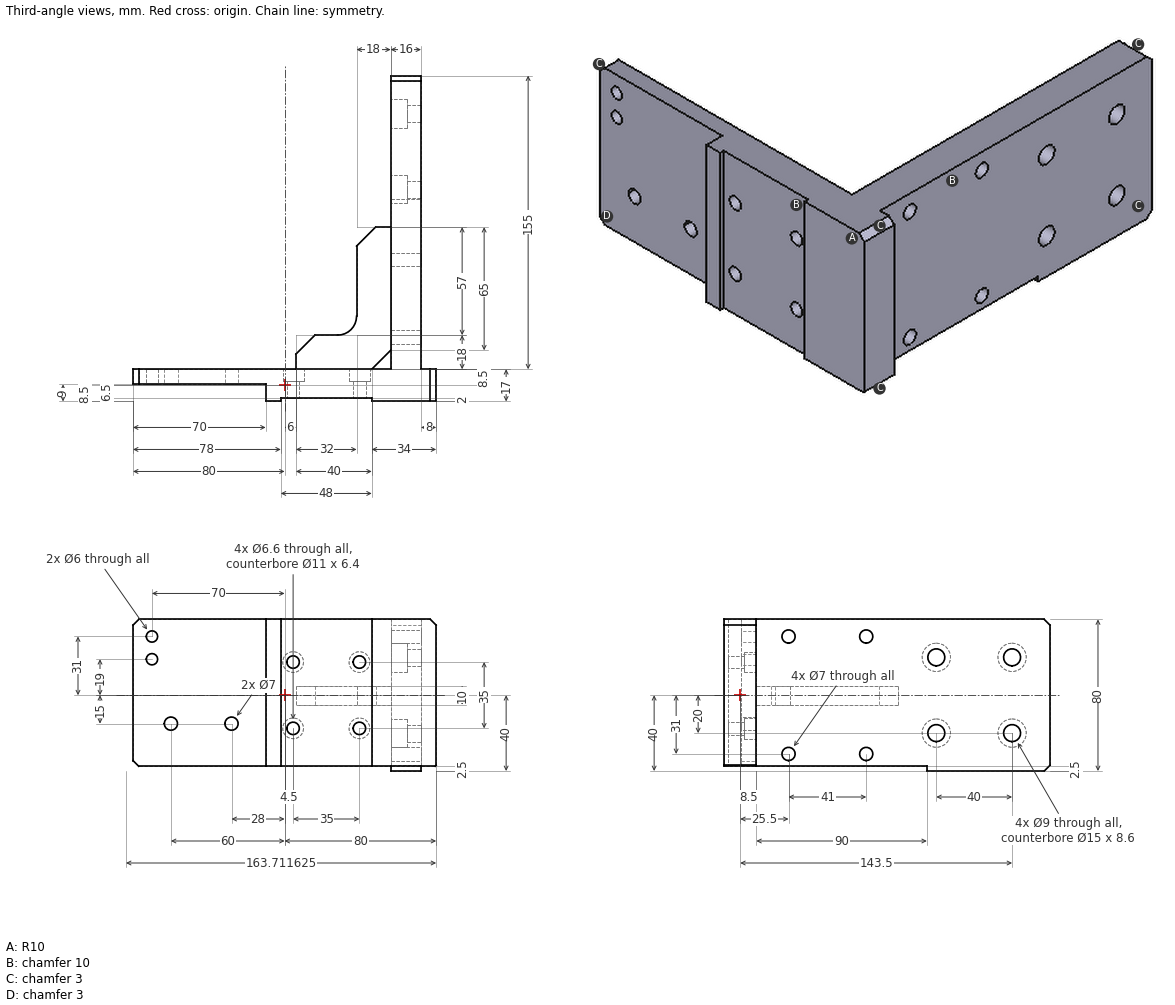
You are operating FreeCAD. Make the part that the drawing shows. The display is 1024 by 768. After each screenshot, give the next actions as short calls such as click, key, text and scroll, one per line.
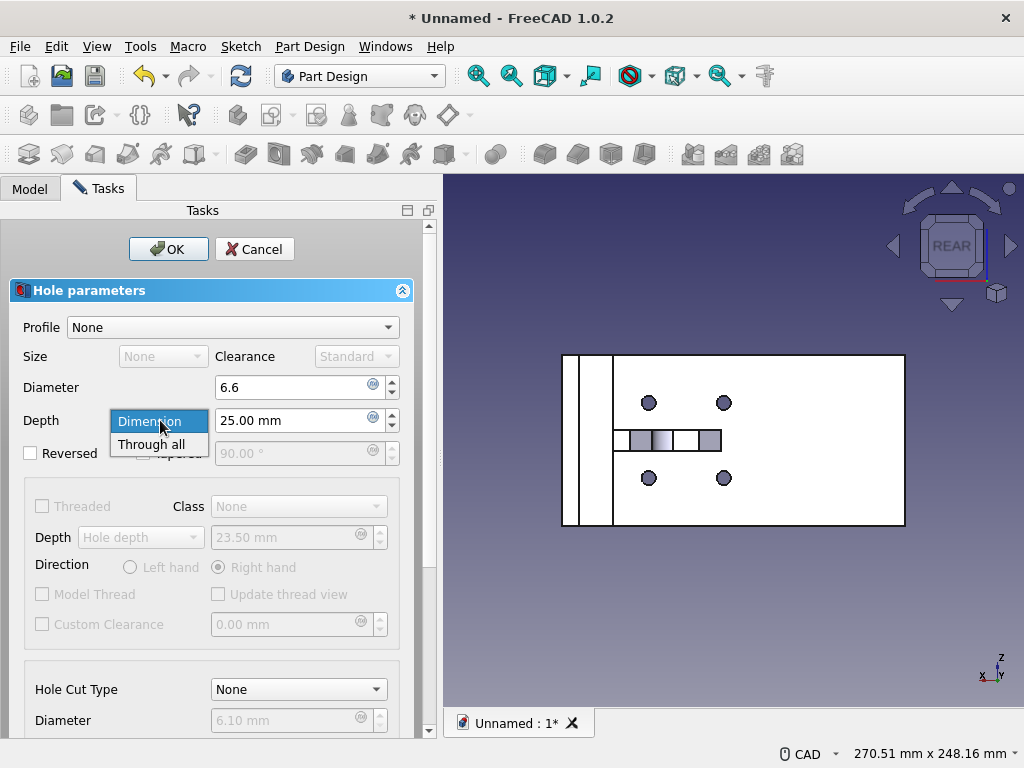
click(158, 444)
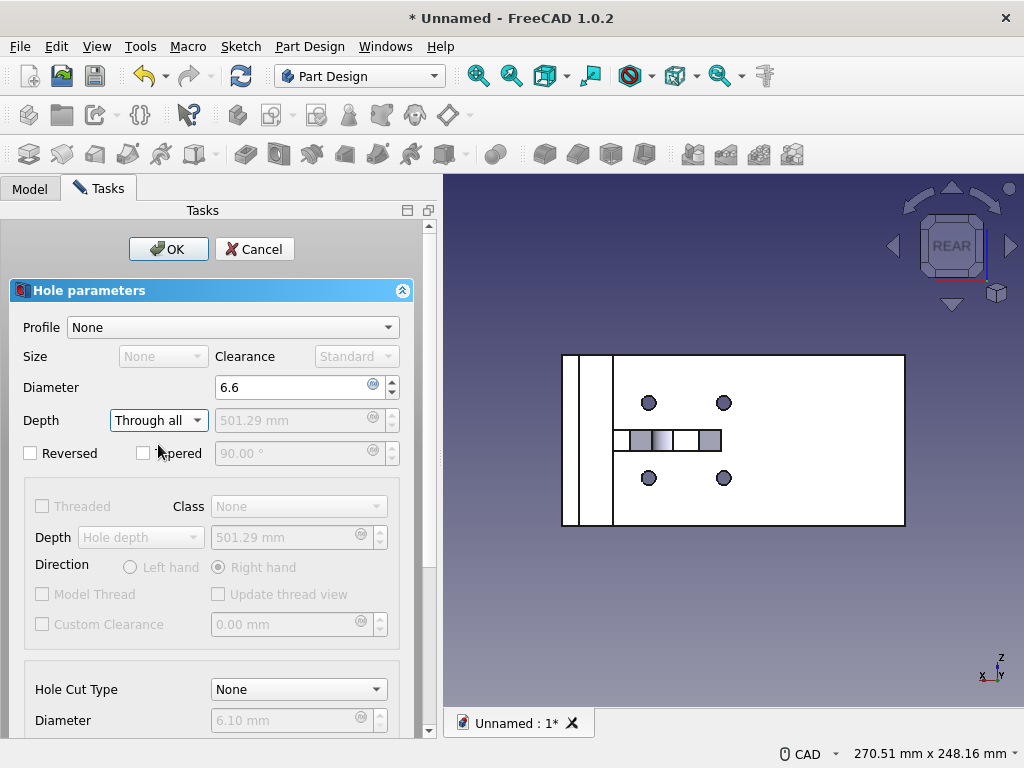
click(300, 690)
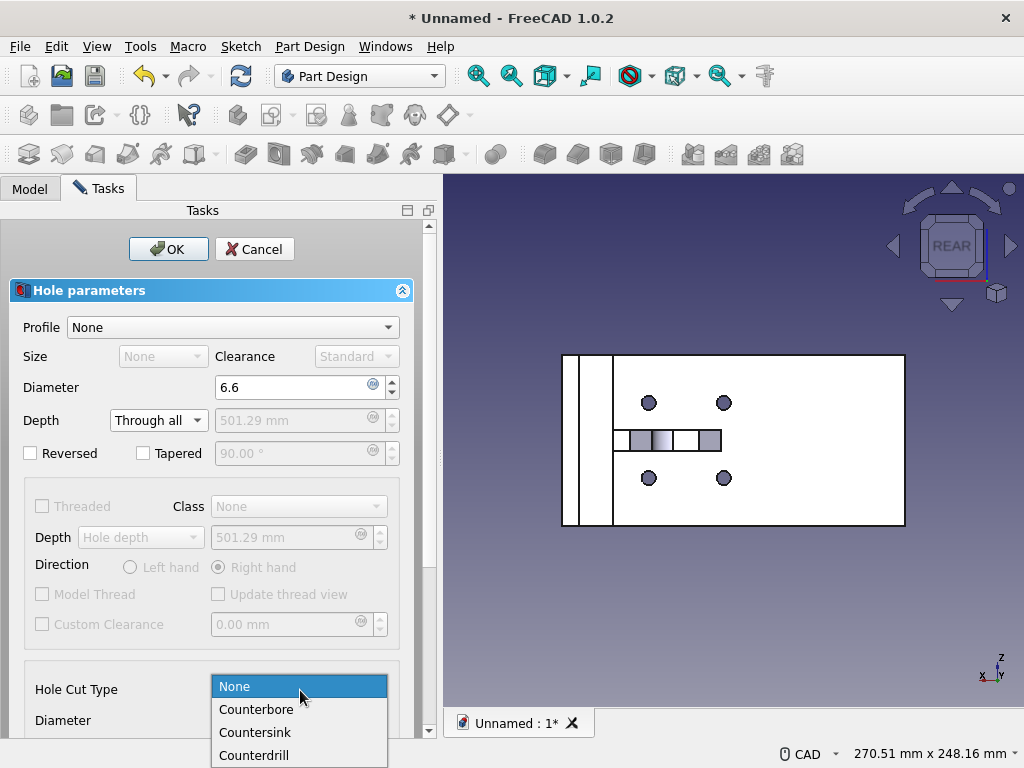
click(298, 710)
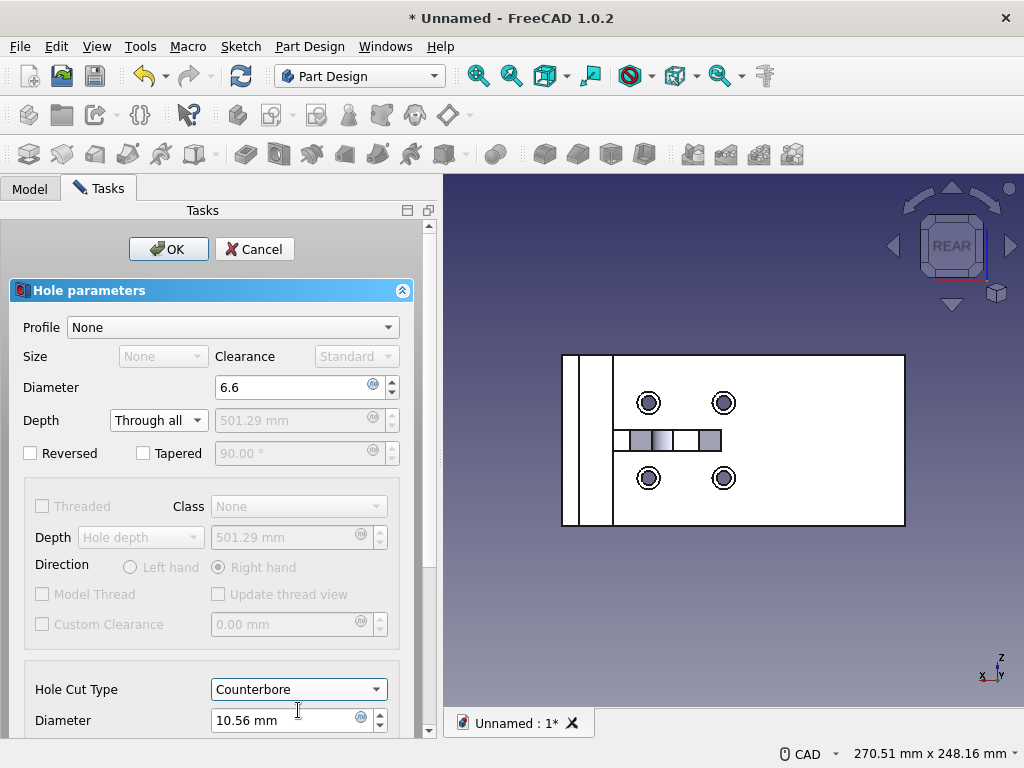
triple_click(292, 720)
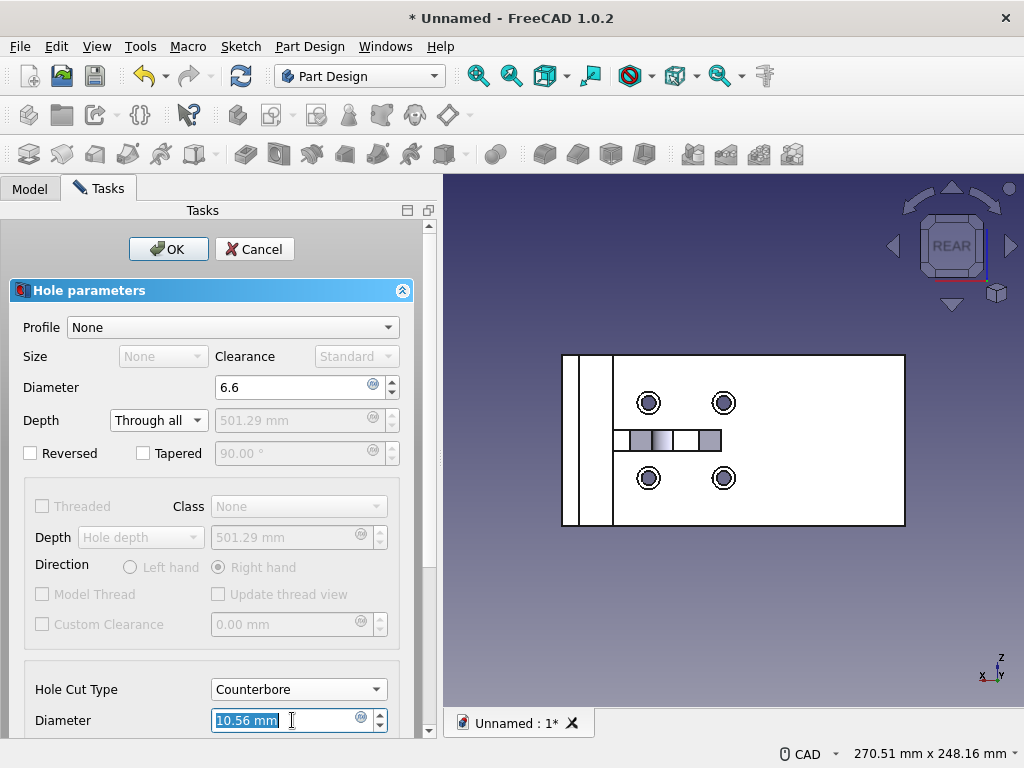
text(11)
key(Tab)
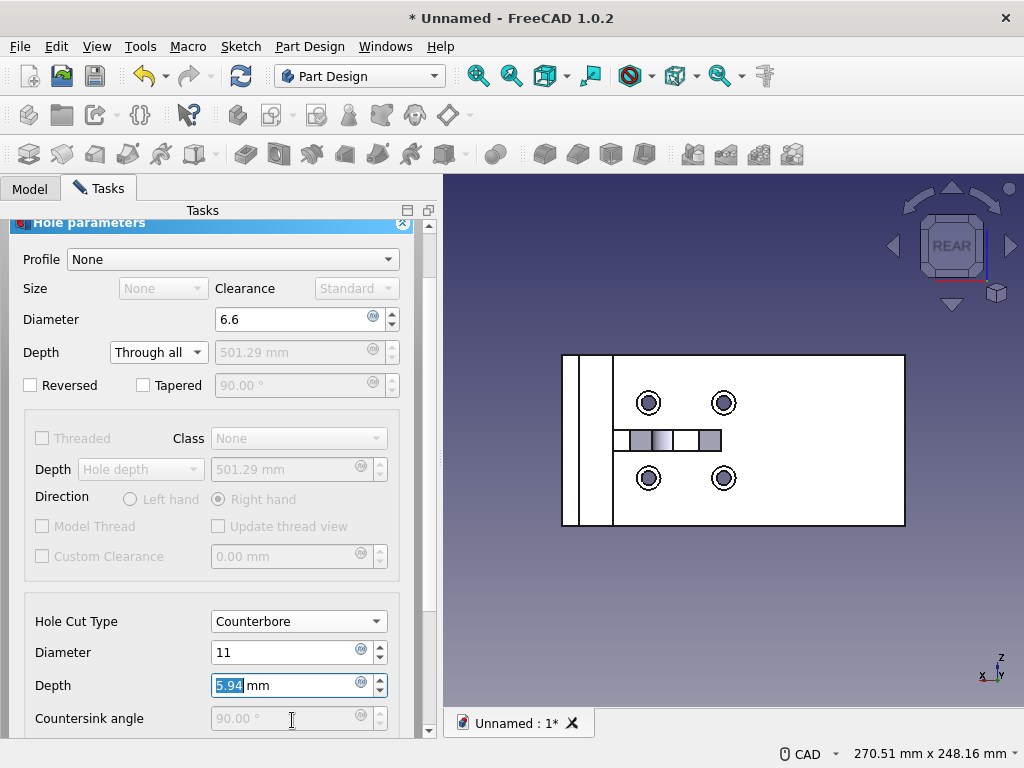
text(6.4)
key(Tab)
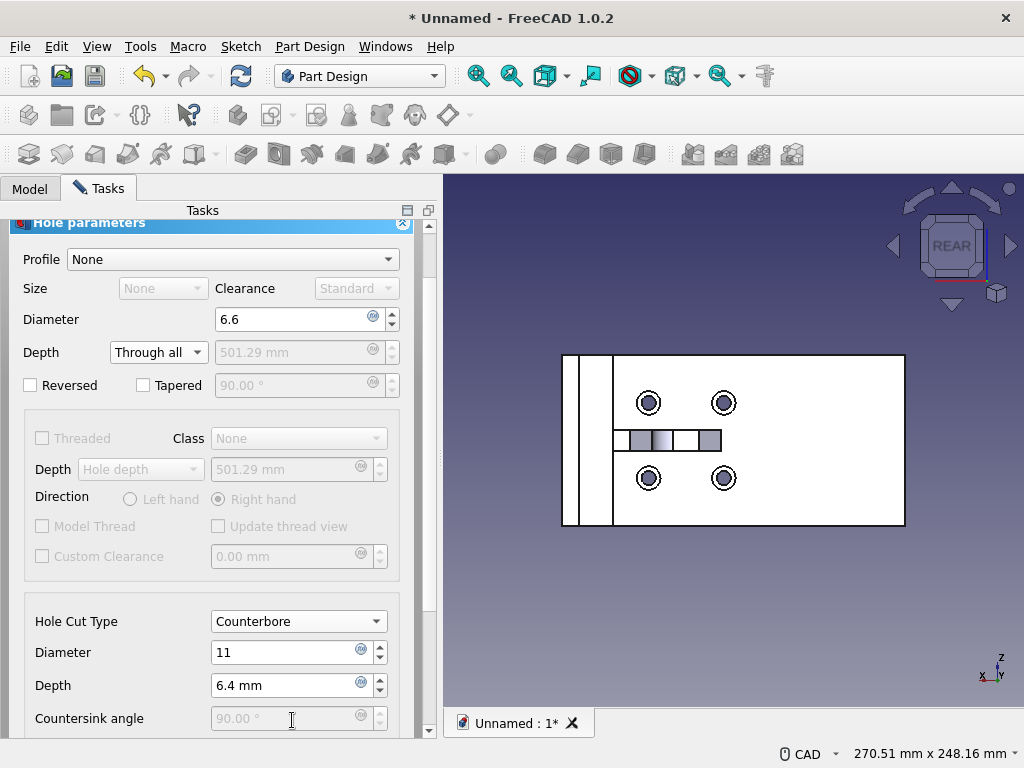
scroll(429, 479, up, 2)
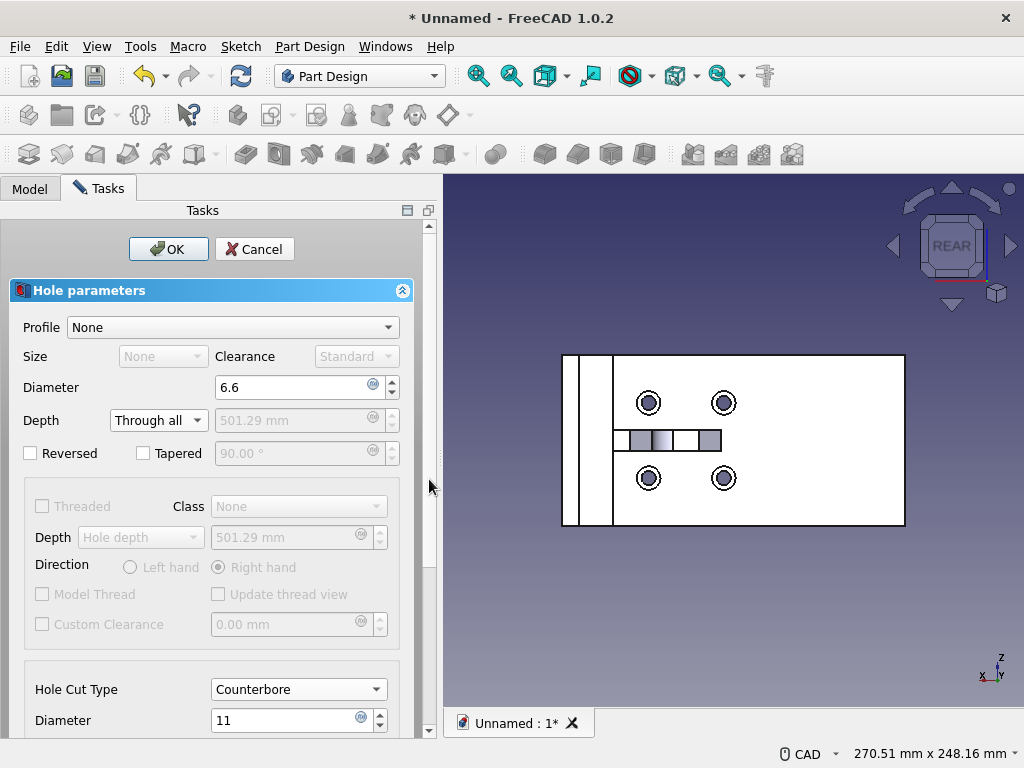
click(169, 249)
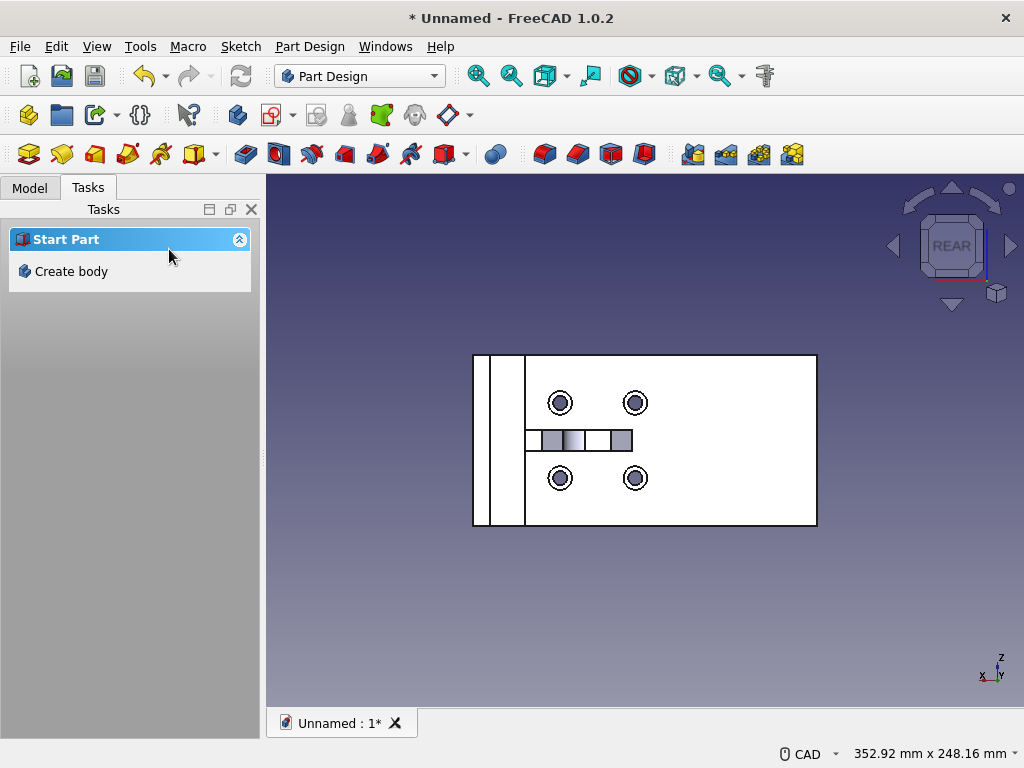
click(508, 354)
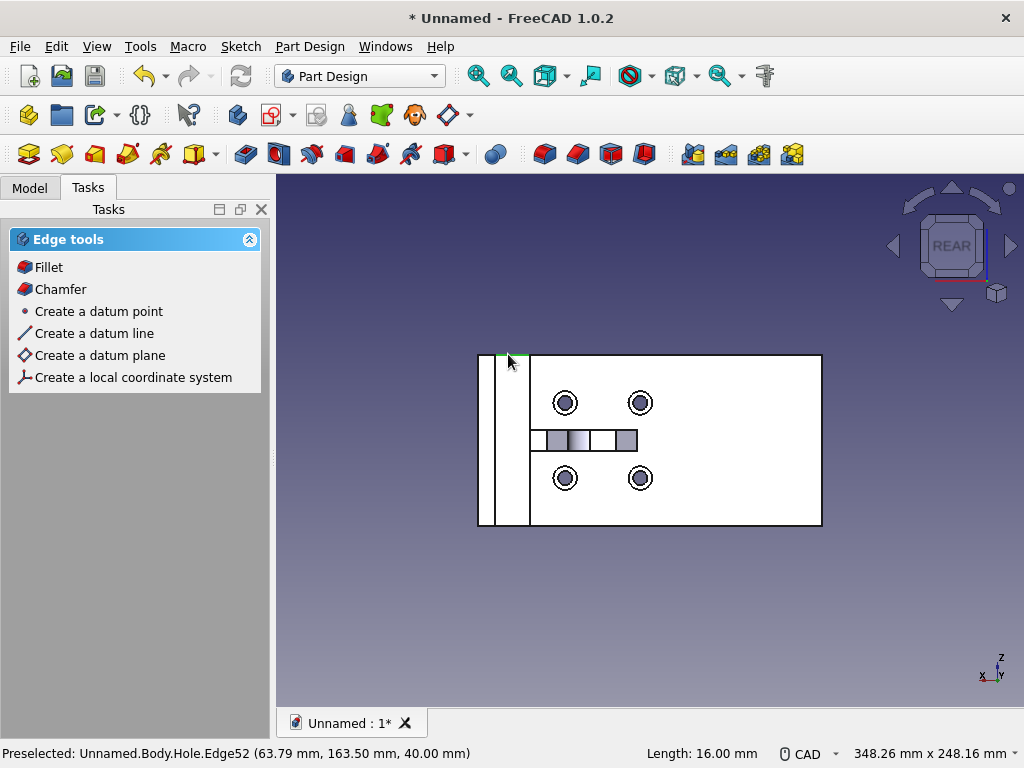
click(513, 525, ctrl)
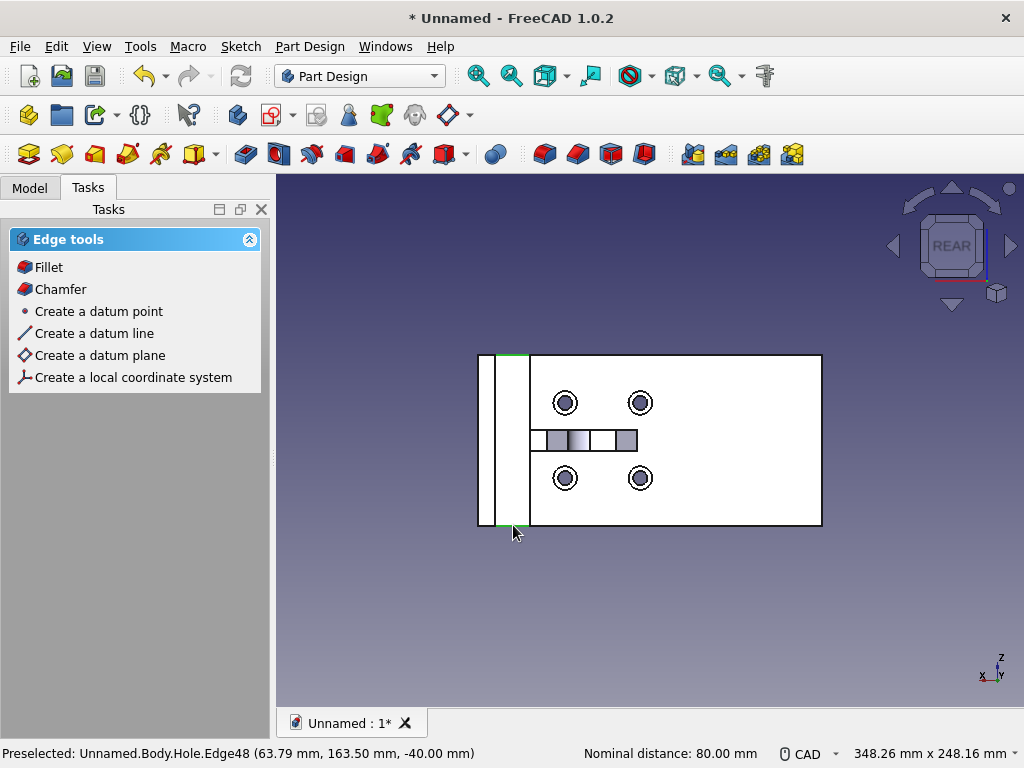
key(0)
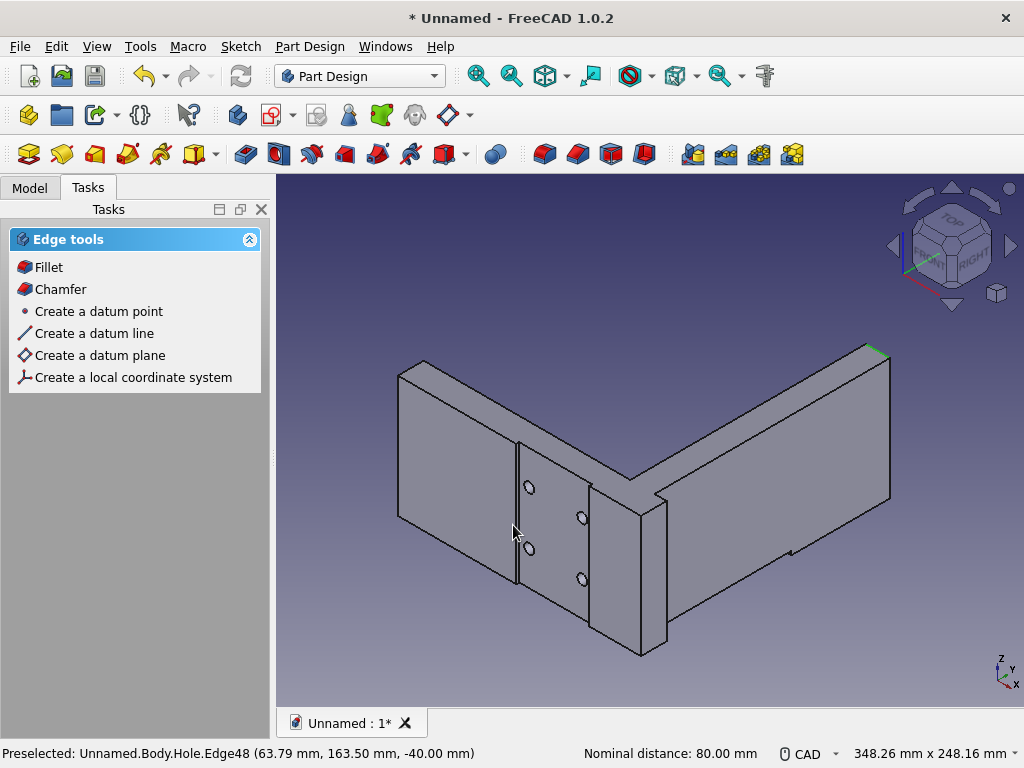
click(654, 507, ctrl)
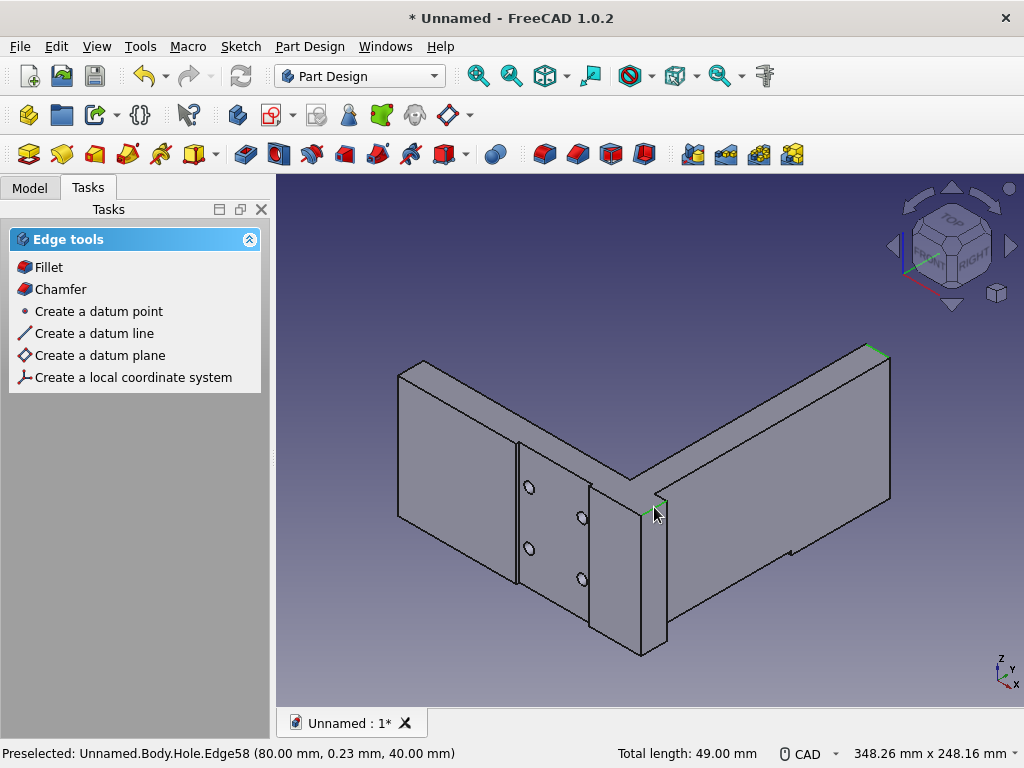
key(2)